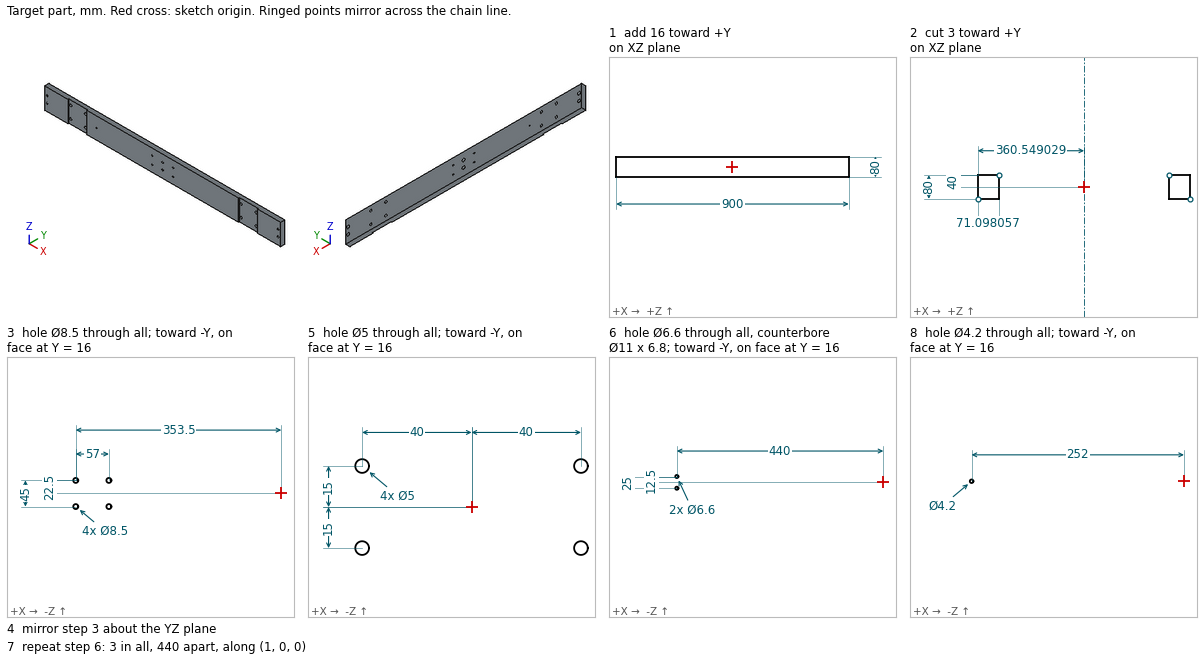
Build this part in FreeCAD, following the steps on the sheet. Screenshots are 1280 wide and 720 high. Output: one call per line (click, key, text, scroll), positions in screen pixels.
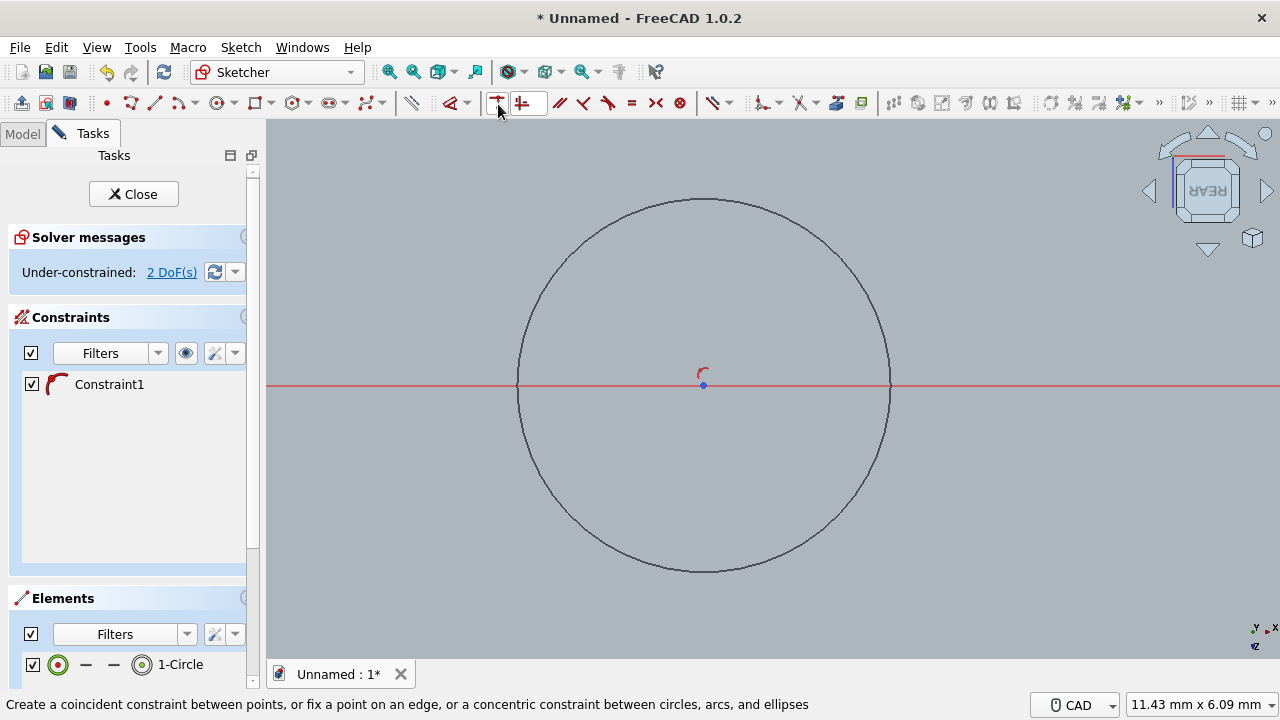
click(450, 104)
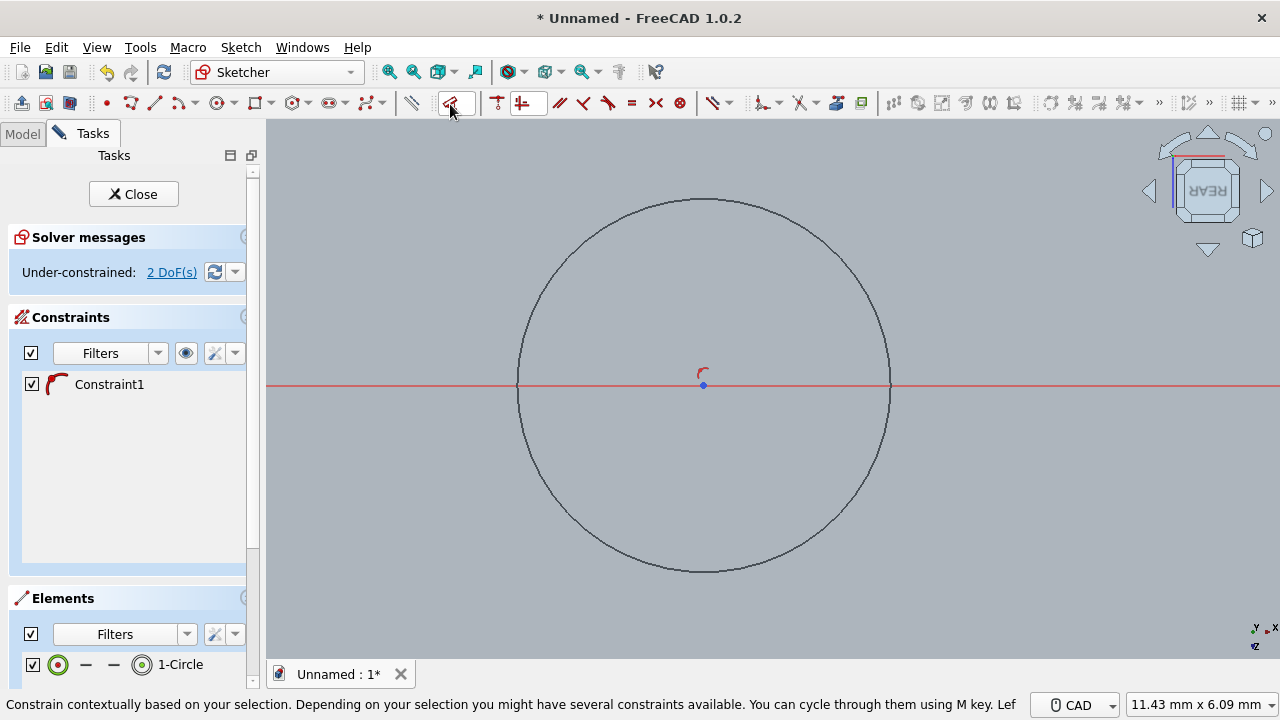
click(836, 253)
click(859, 230)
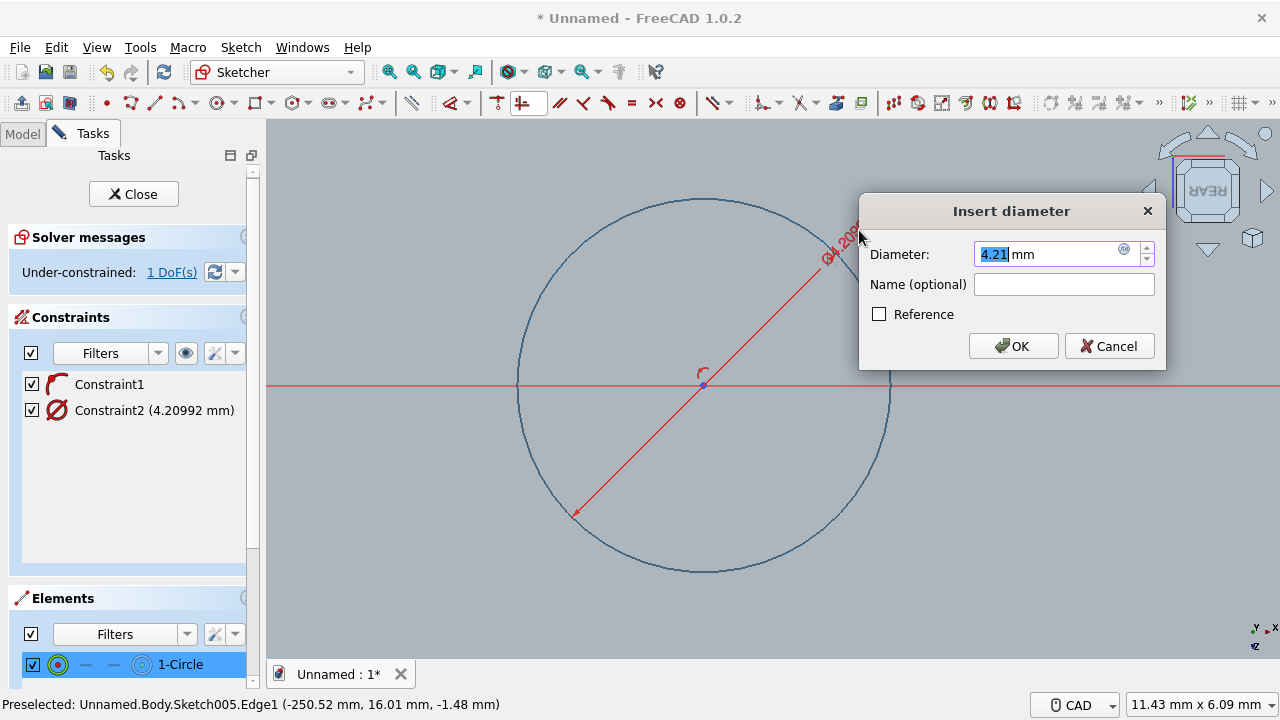
text(4.2)
key(Return)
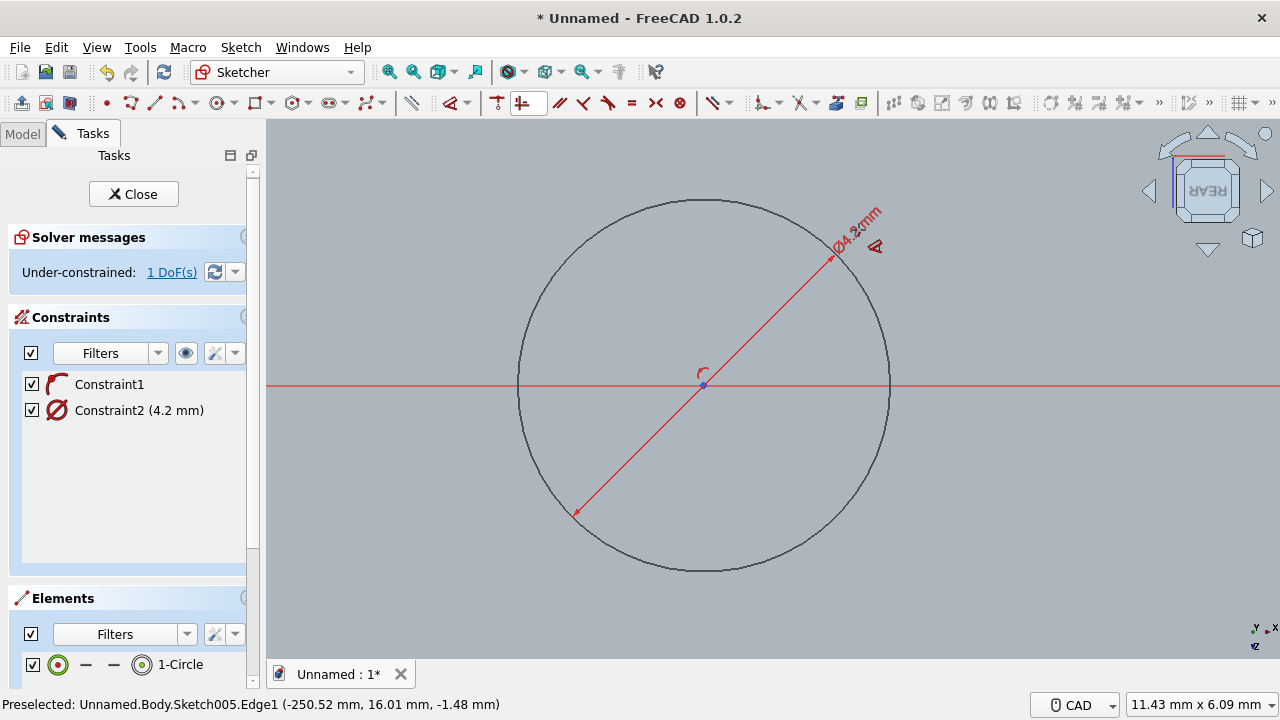
click(704, 386)
click(909, 420)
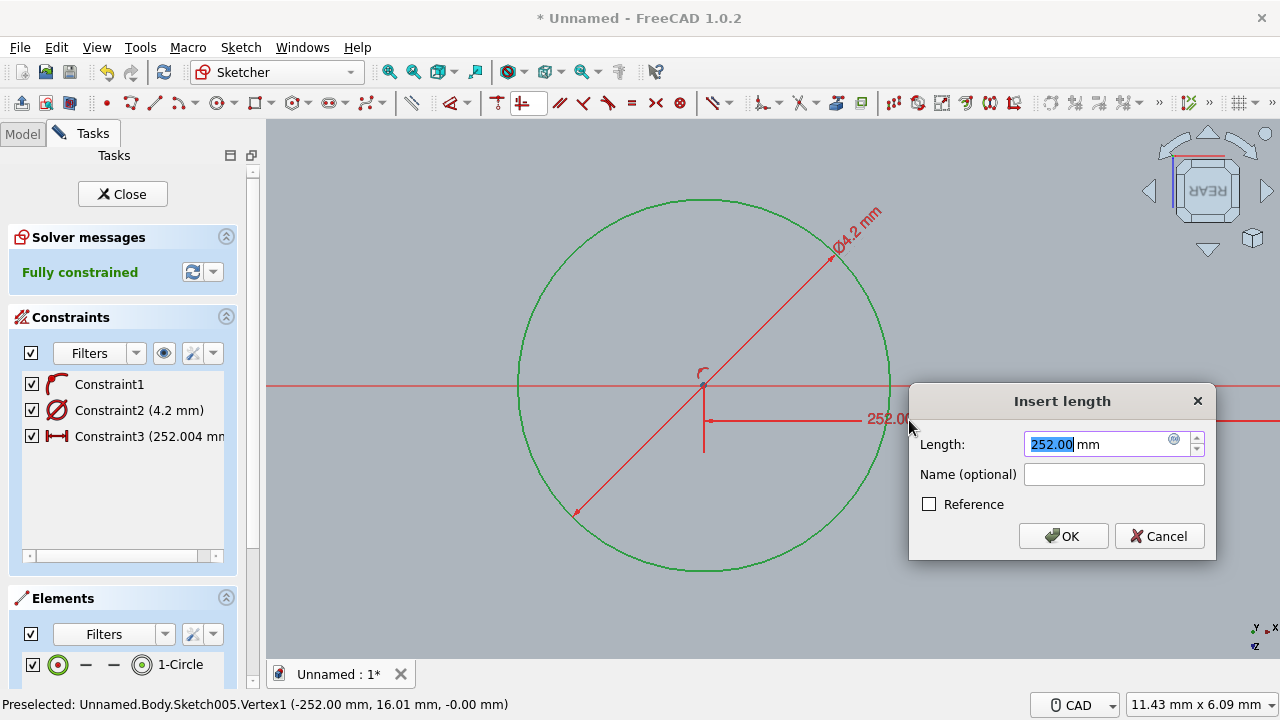
text(252)
key(Return)
key(Escape)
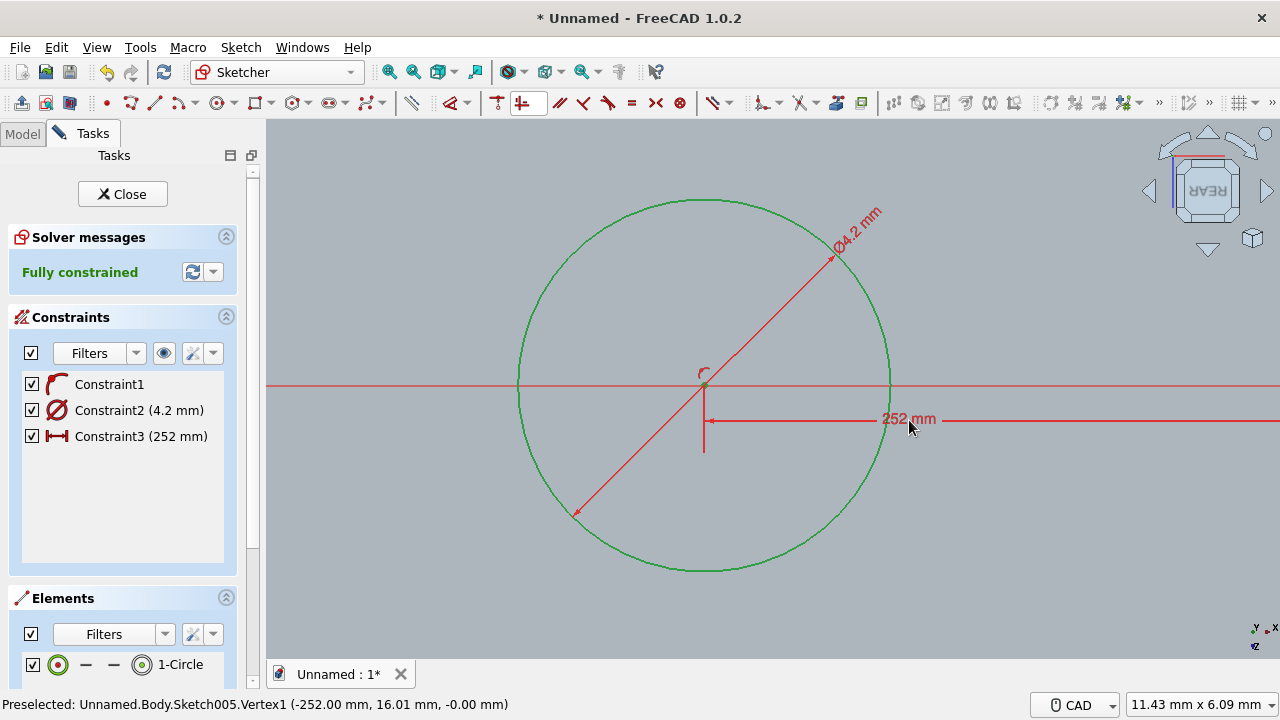
click(123, 194)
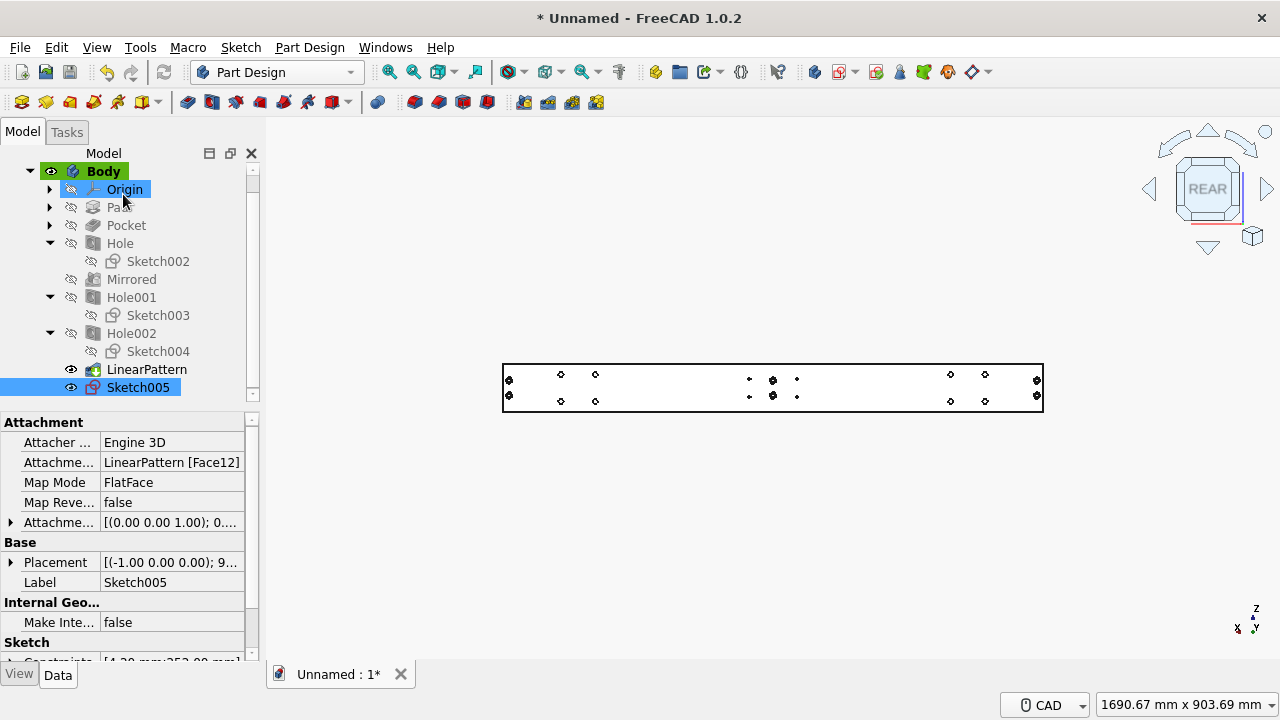
click(212, 102)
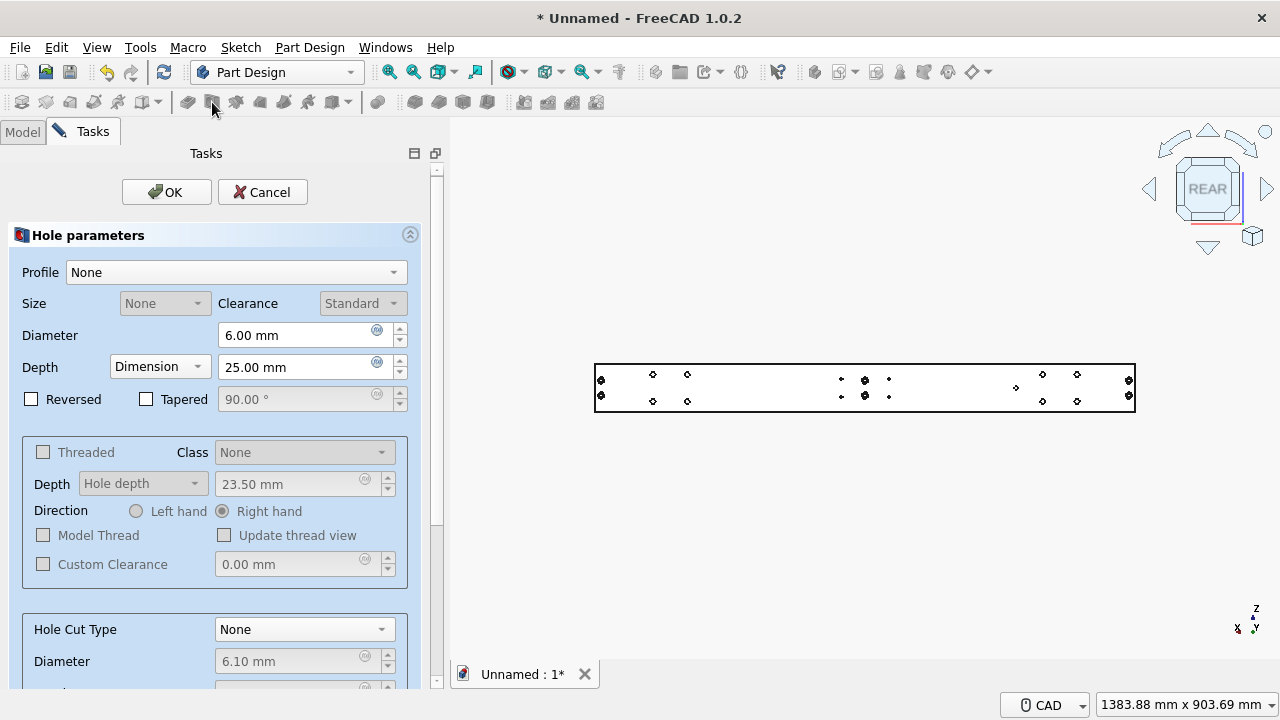
triple_click(305, 335)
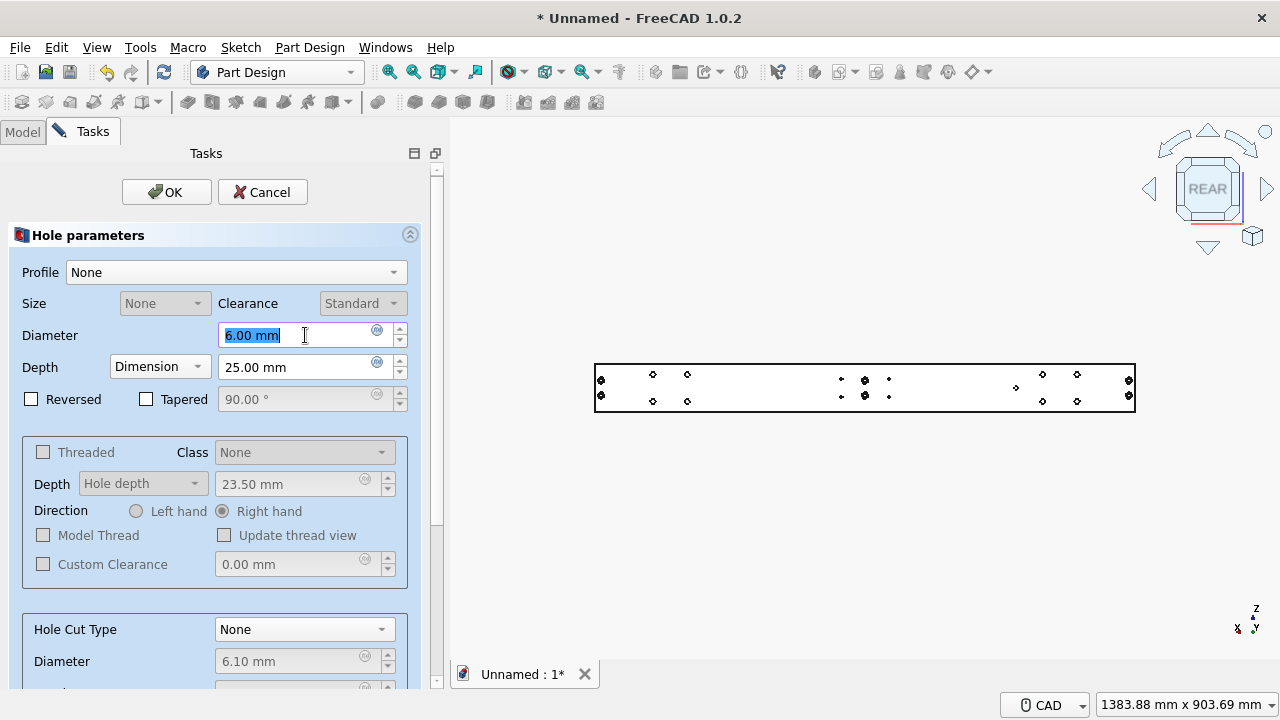
text(4.2)
key(Tab)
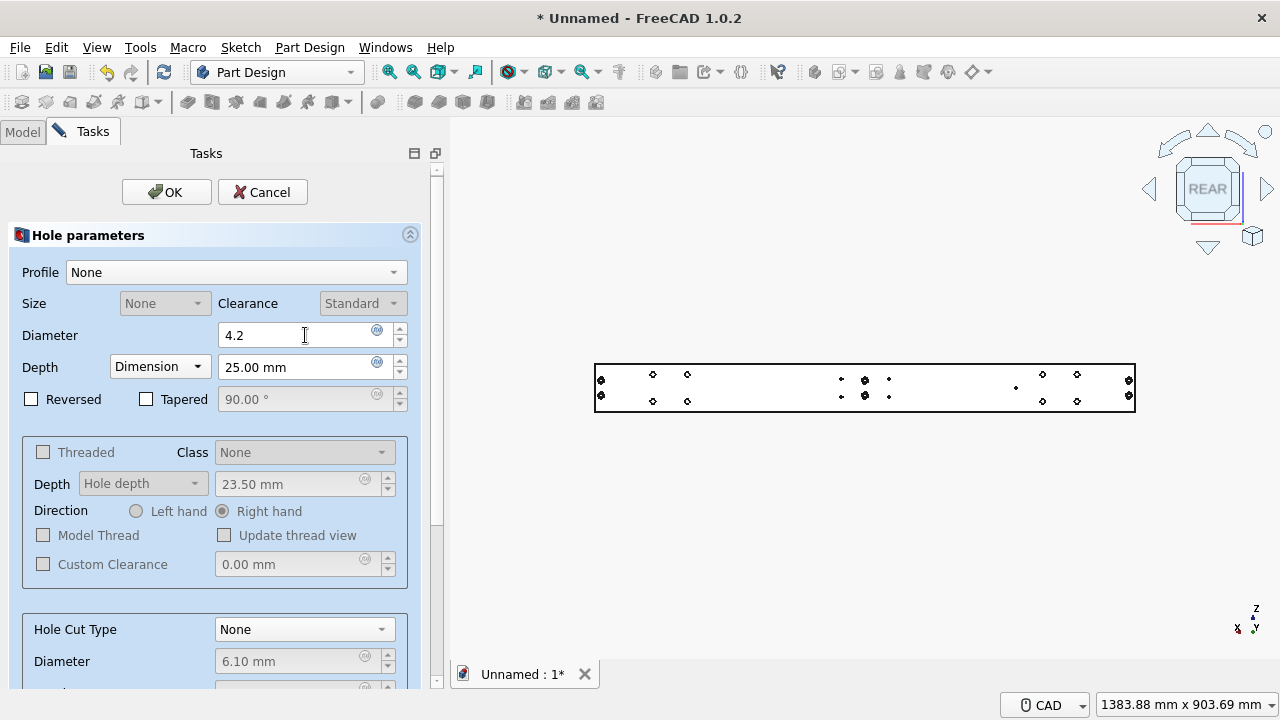
click(161, 366)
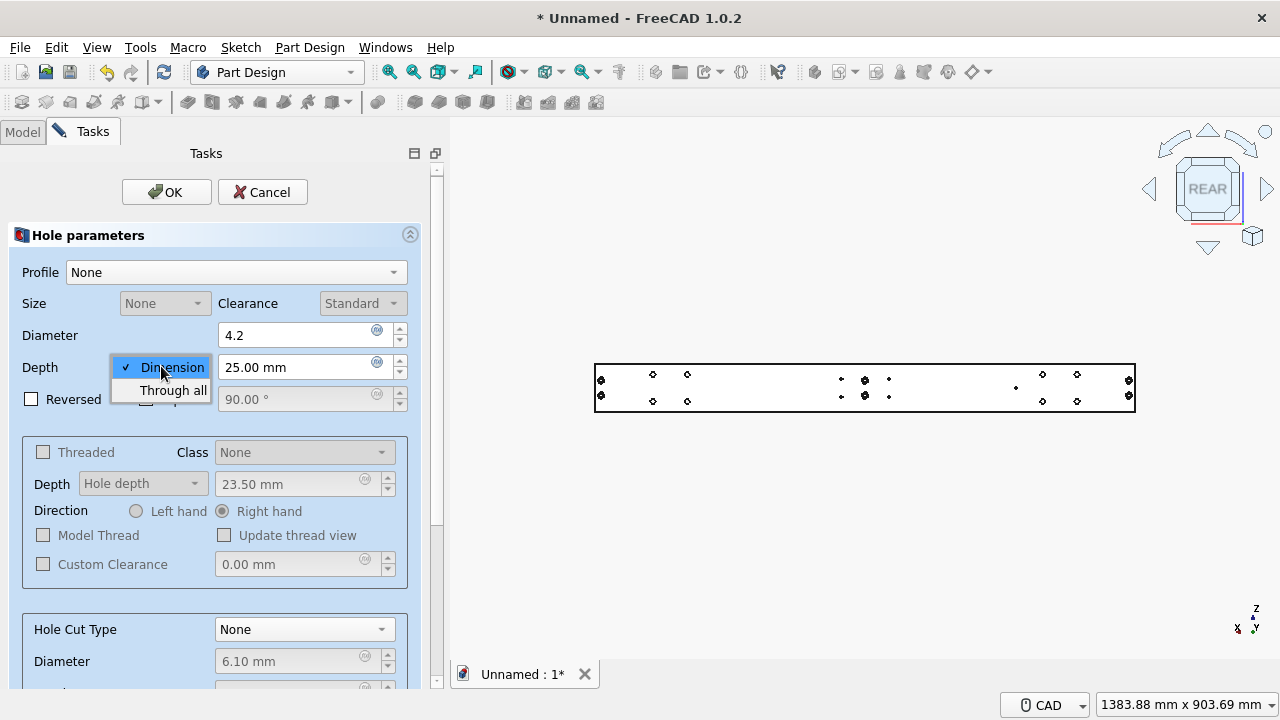
click(160, 390)